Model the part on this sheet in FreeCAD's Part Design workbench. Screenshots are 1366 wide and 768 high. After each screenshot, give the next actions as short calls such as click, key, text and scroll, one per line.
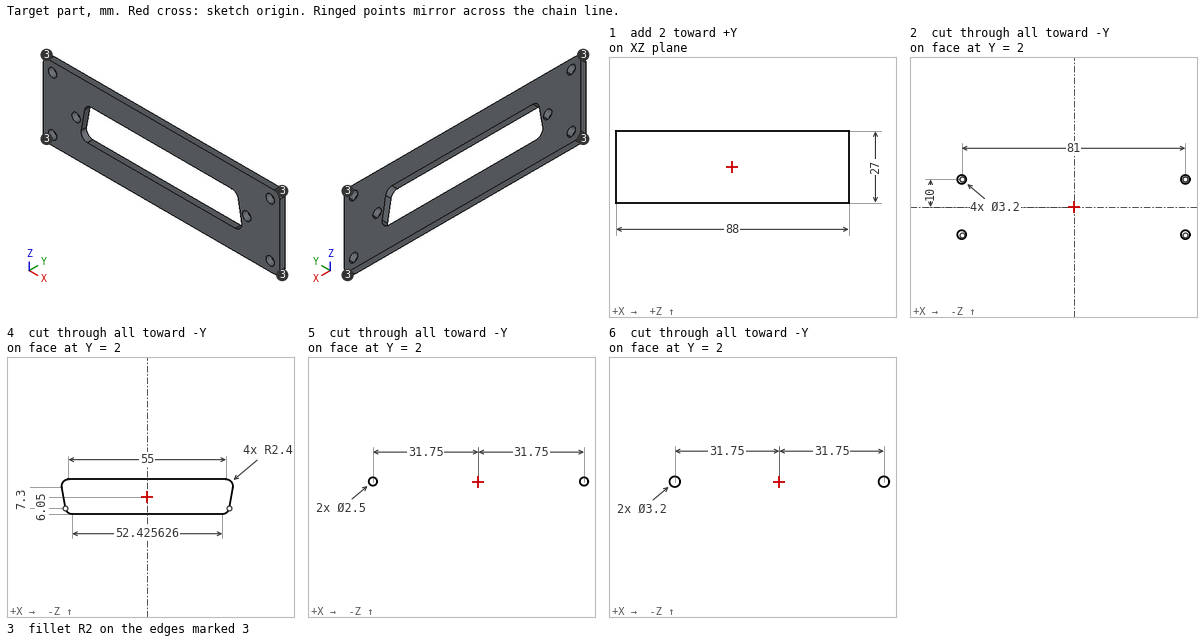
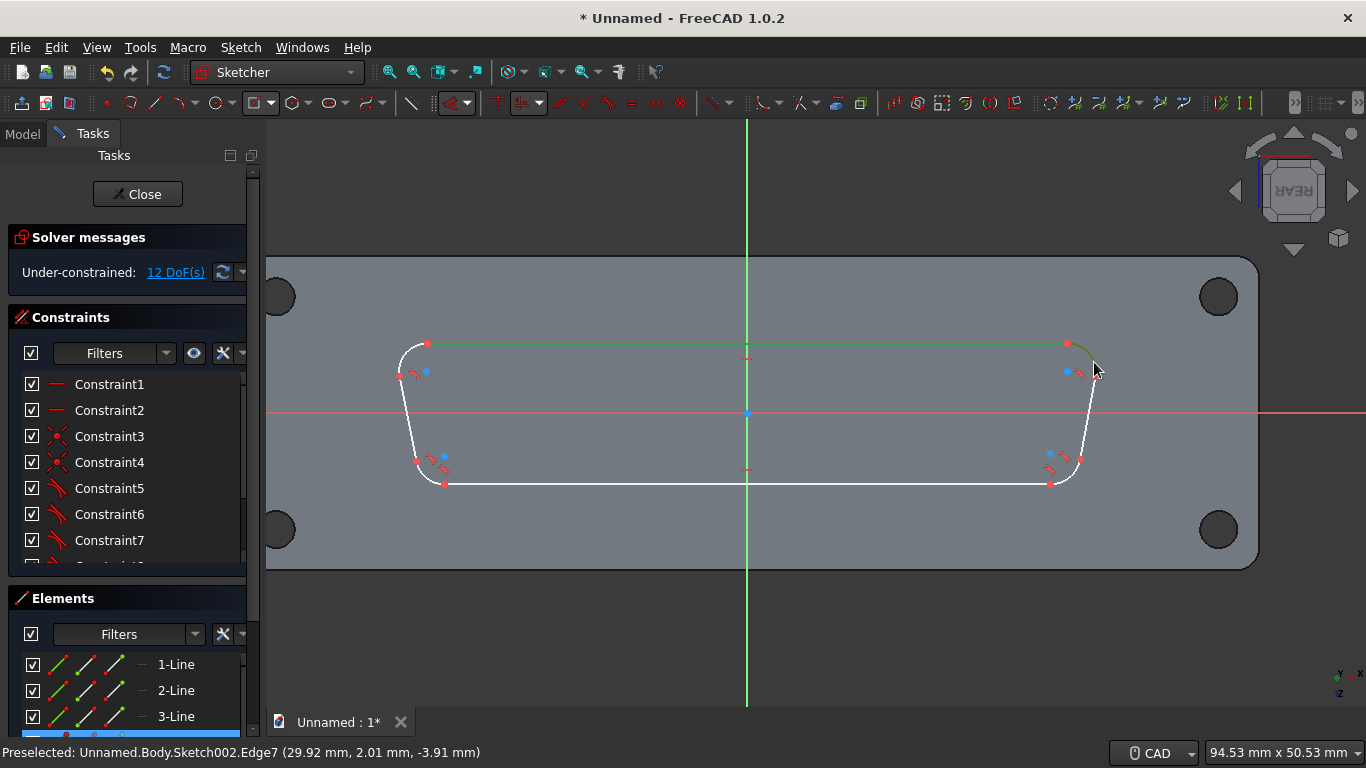
key(t)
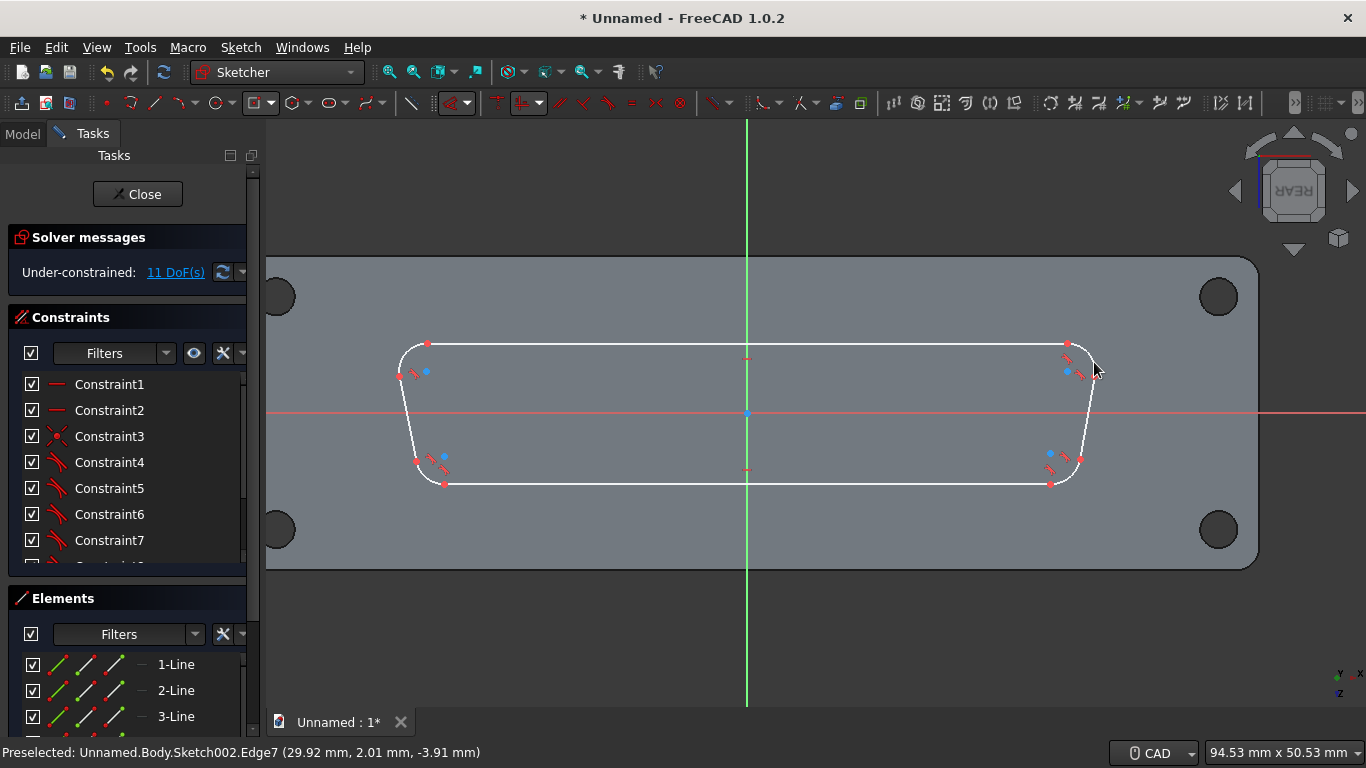
click(875, 344)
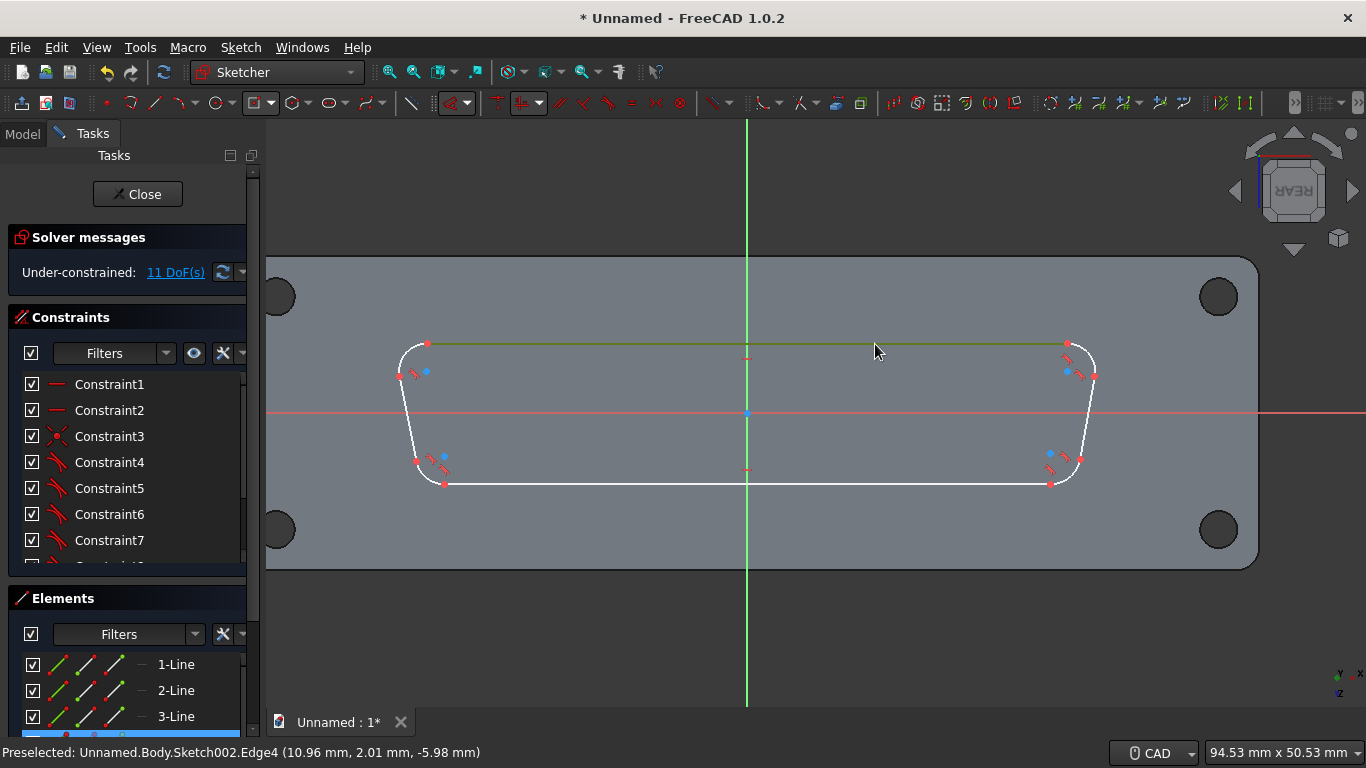
click(413, 347)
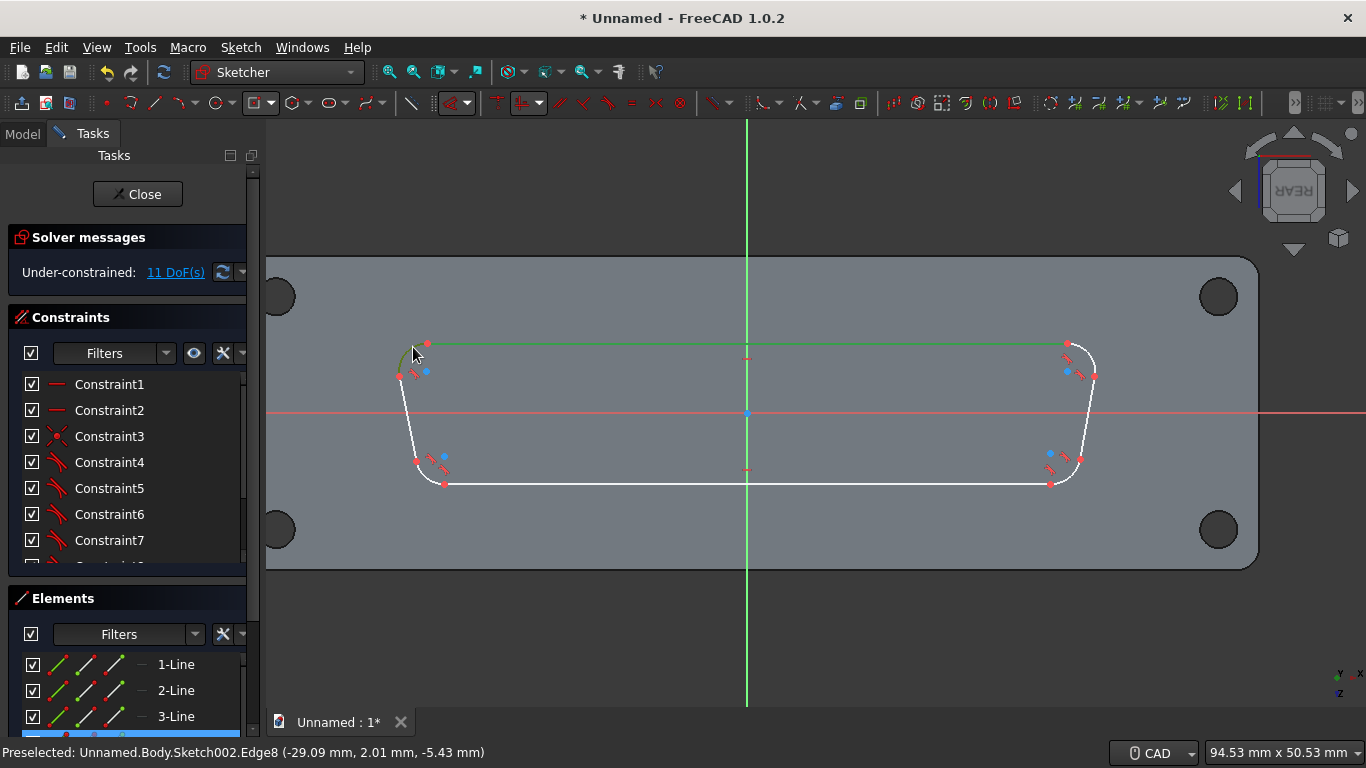
click(608, 104)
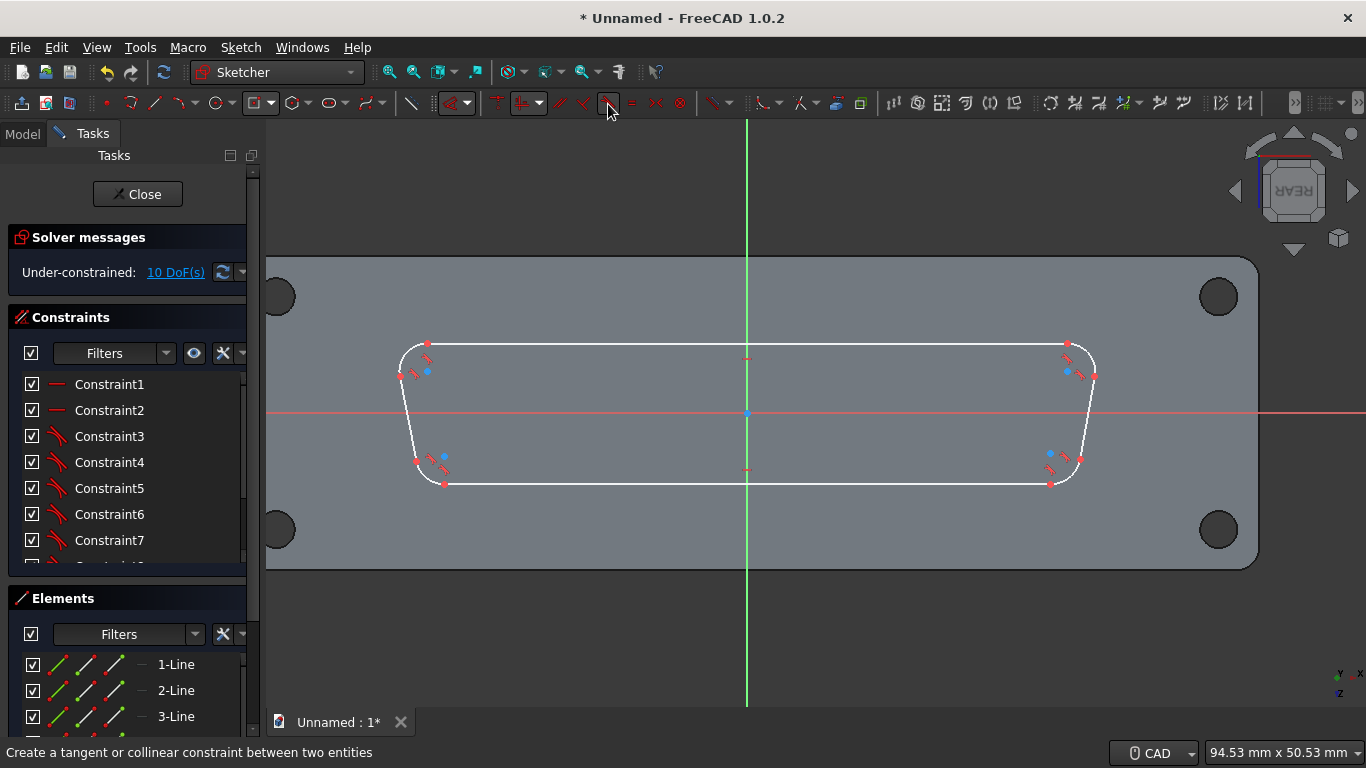
click(421, 472)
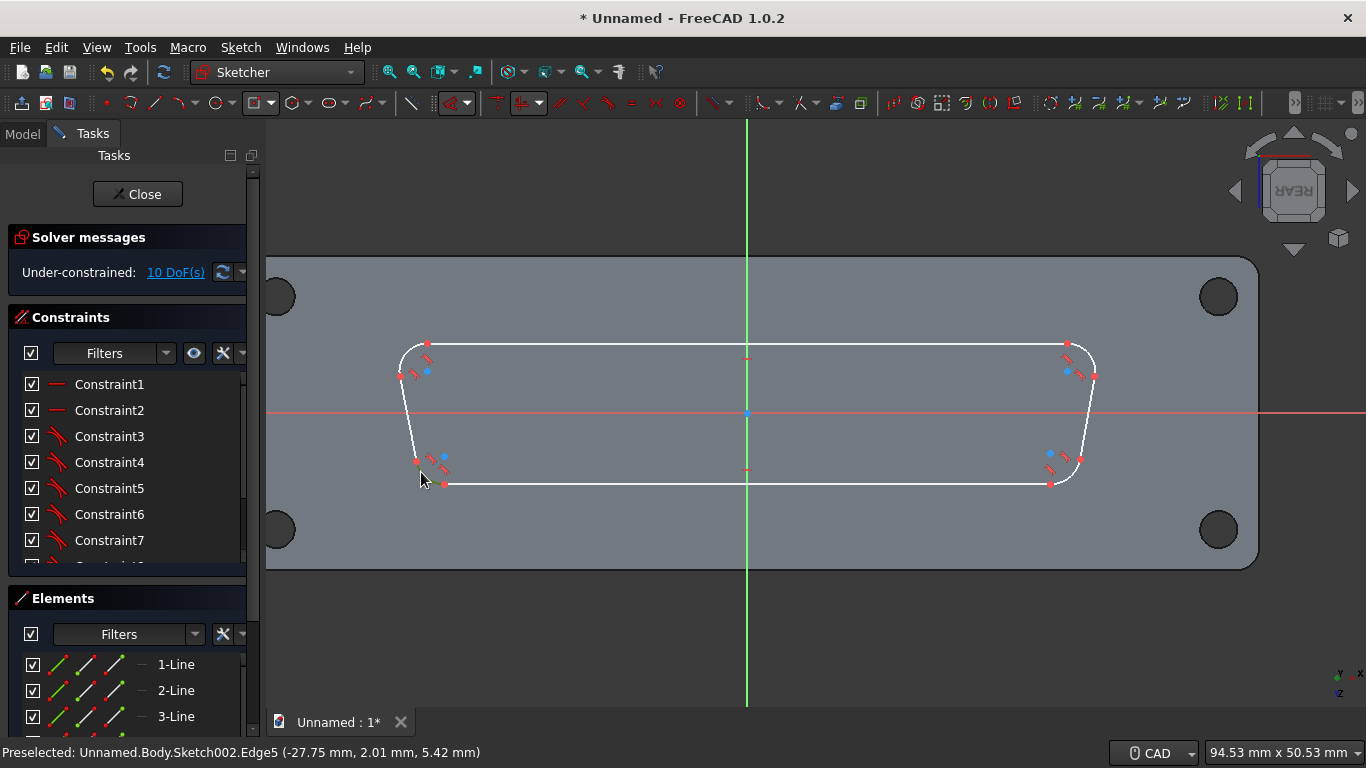
click(1063, 482)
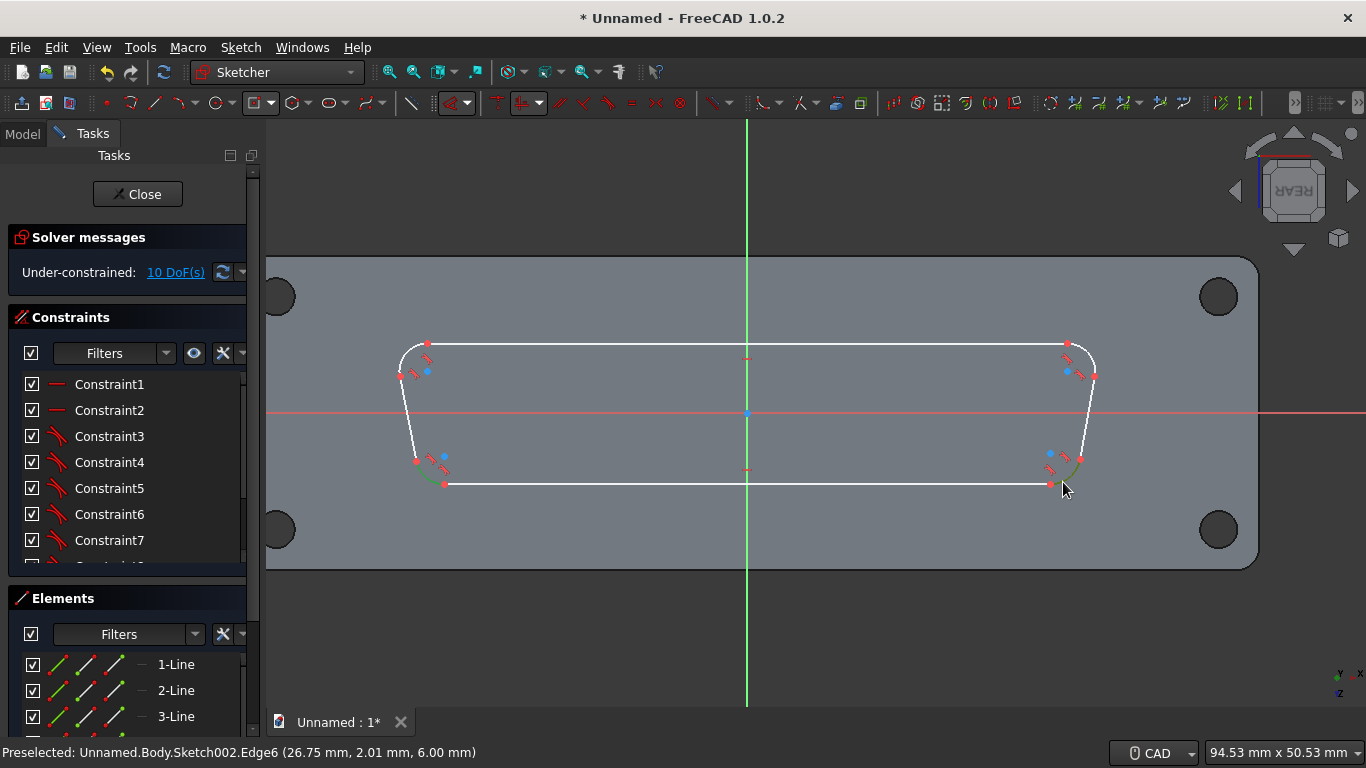
click(1094, 362)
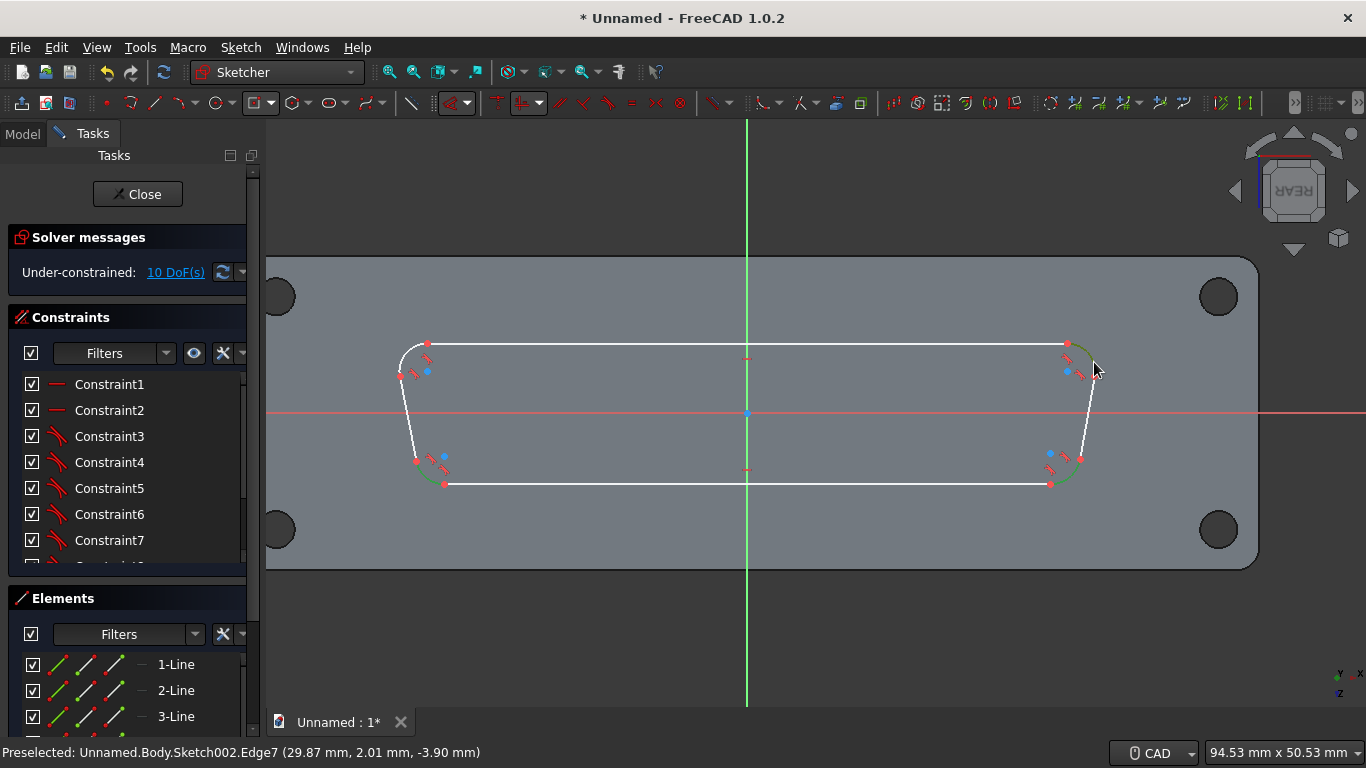
click(413, 347)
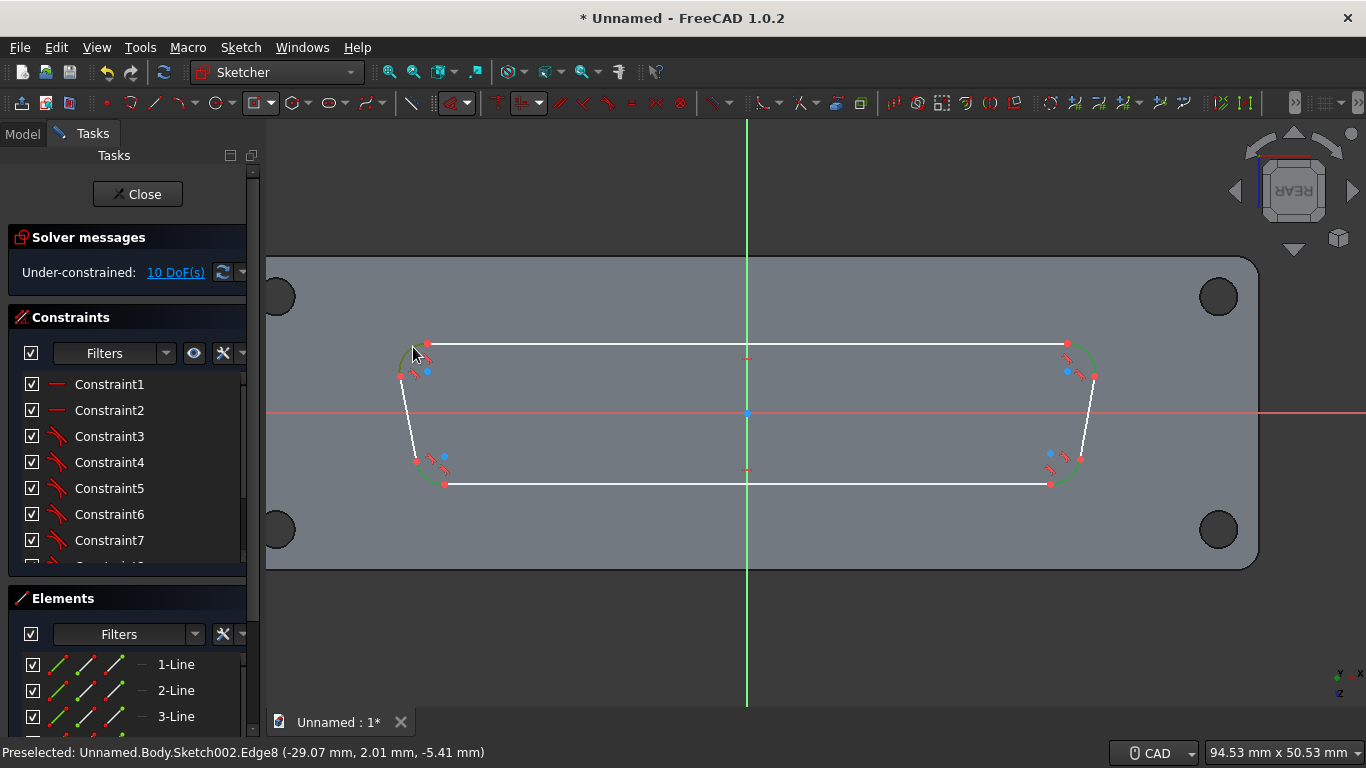
click(632, 104)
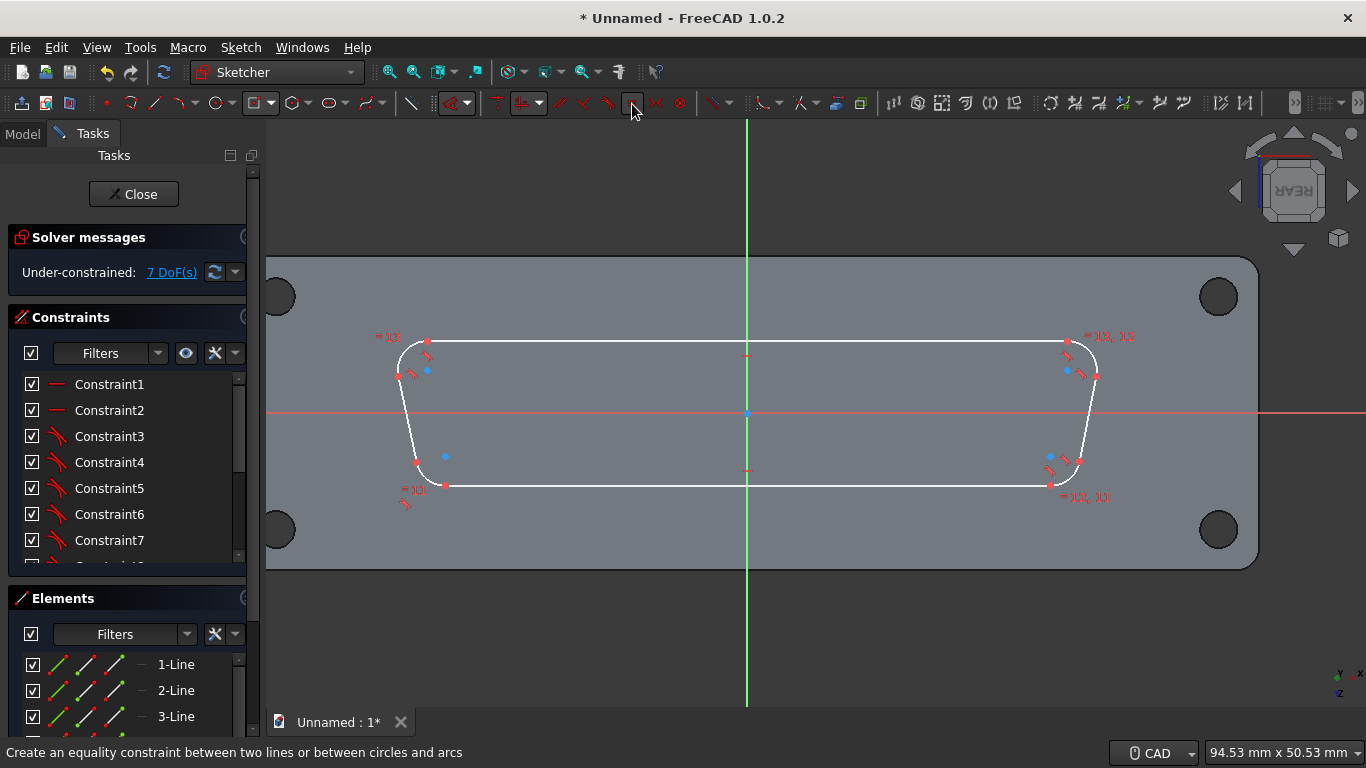
click(417, 462)